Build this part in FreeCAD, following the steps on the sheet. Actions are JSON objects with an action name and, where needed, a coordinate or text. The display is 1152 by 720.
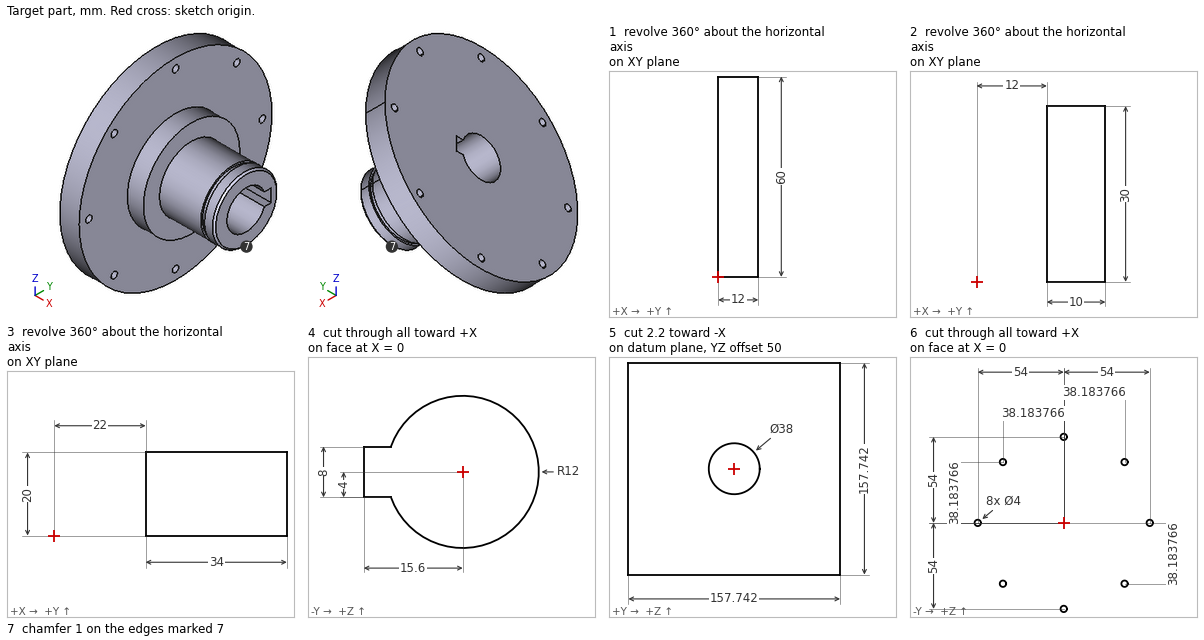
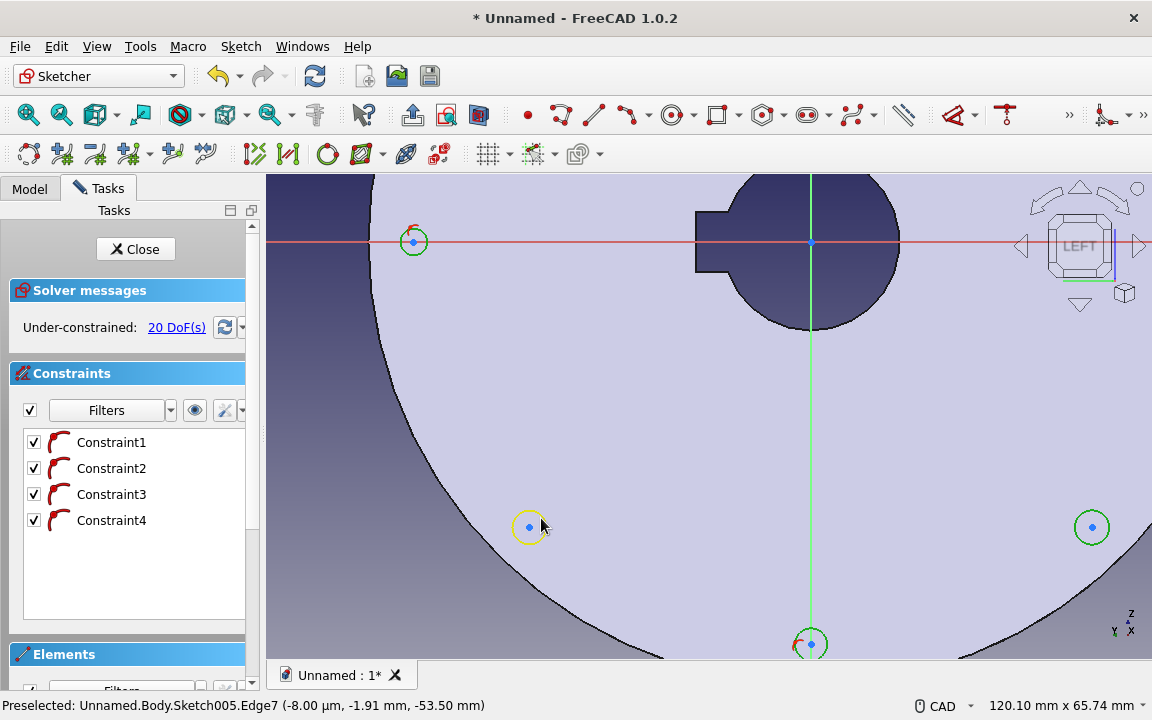
{"action": "left_click", "coordinate": [541, 516]}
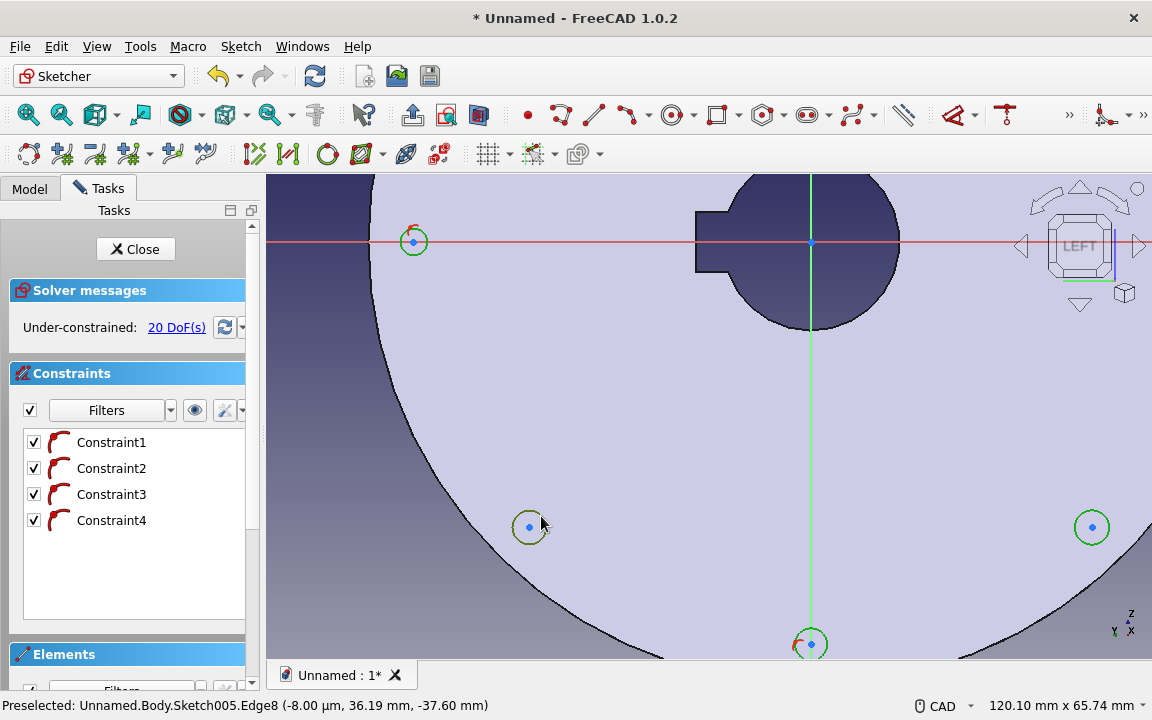
{"action": "key", "text": "e"}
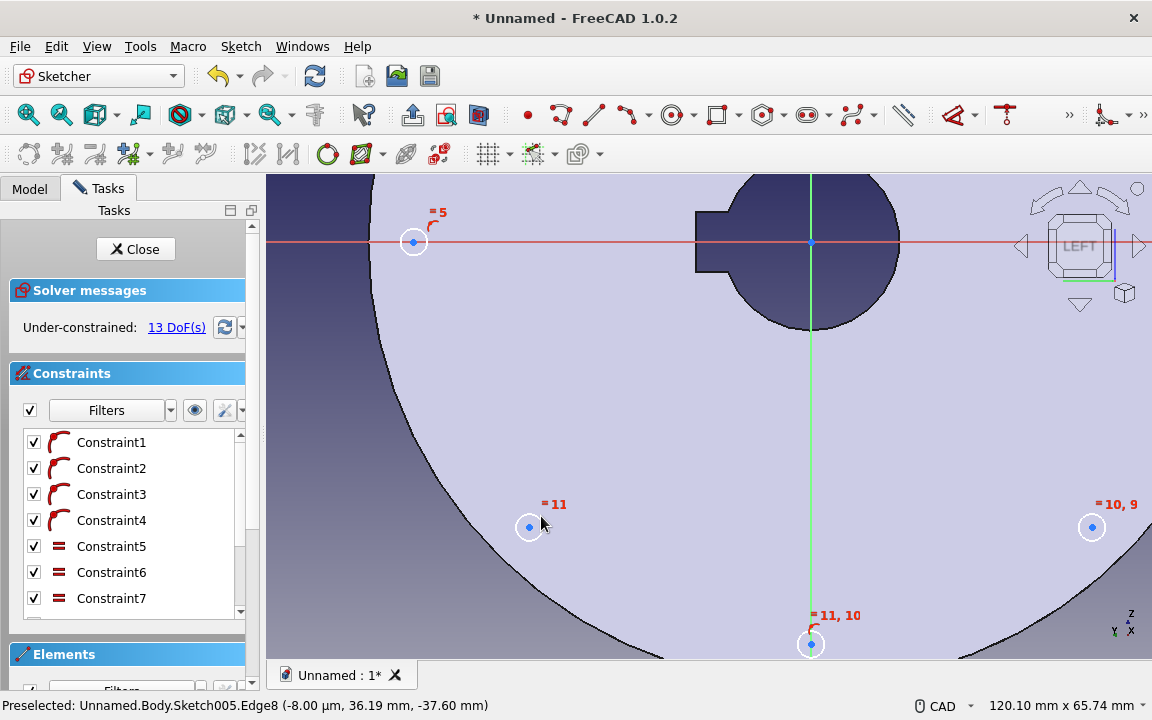
{"action": "scroll", "coordinate": [541, 518], "scroll_direction": "down", "scroll_amount": 5}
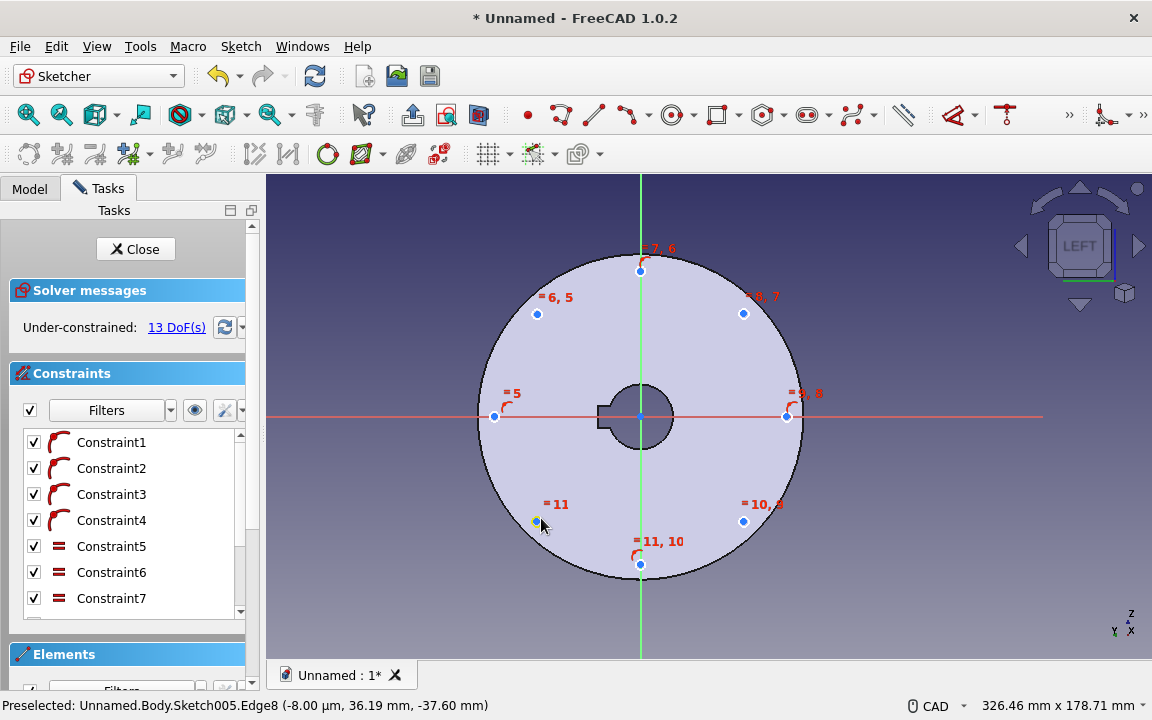
{"action": "left_click", "coordinate": [537, 314]}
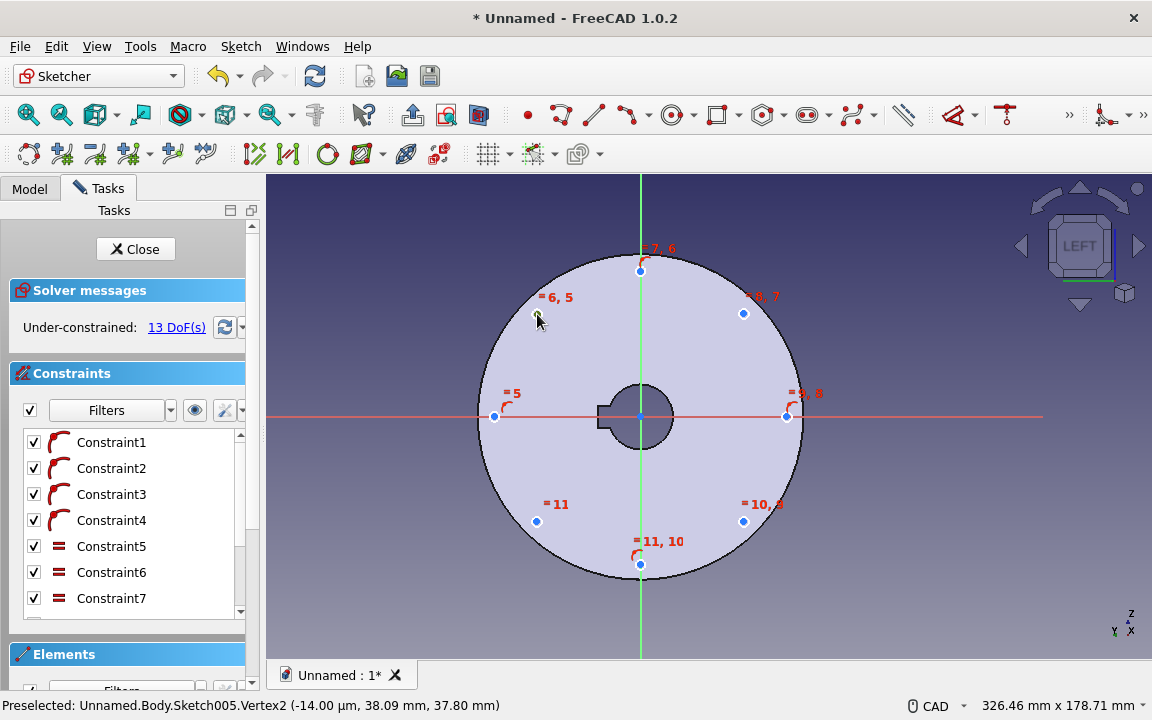
{"action": "left_click", "coordinate": [744, 314]}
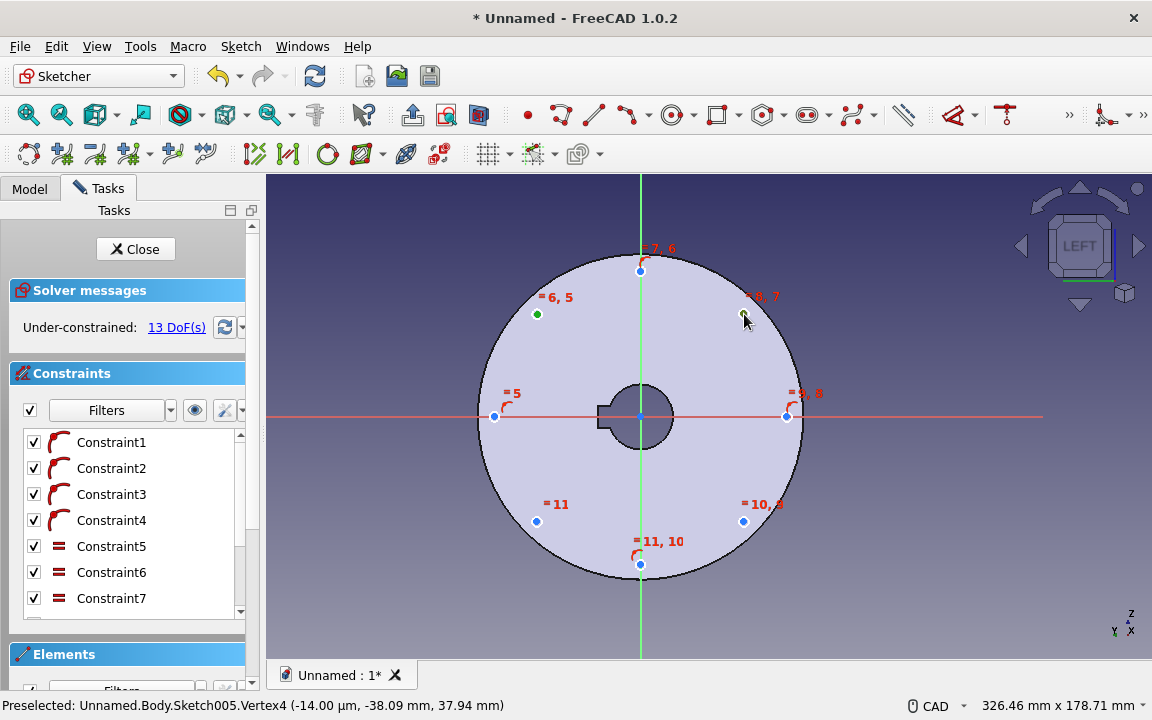
{"action": "key", "text": "h"}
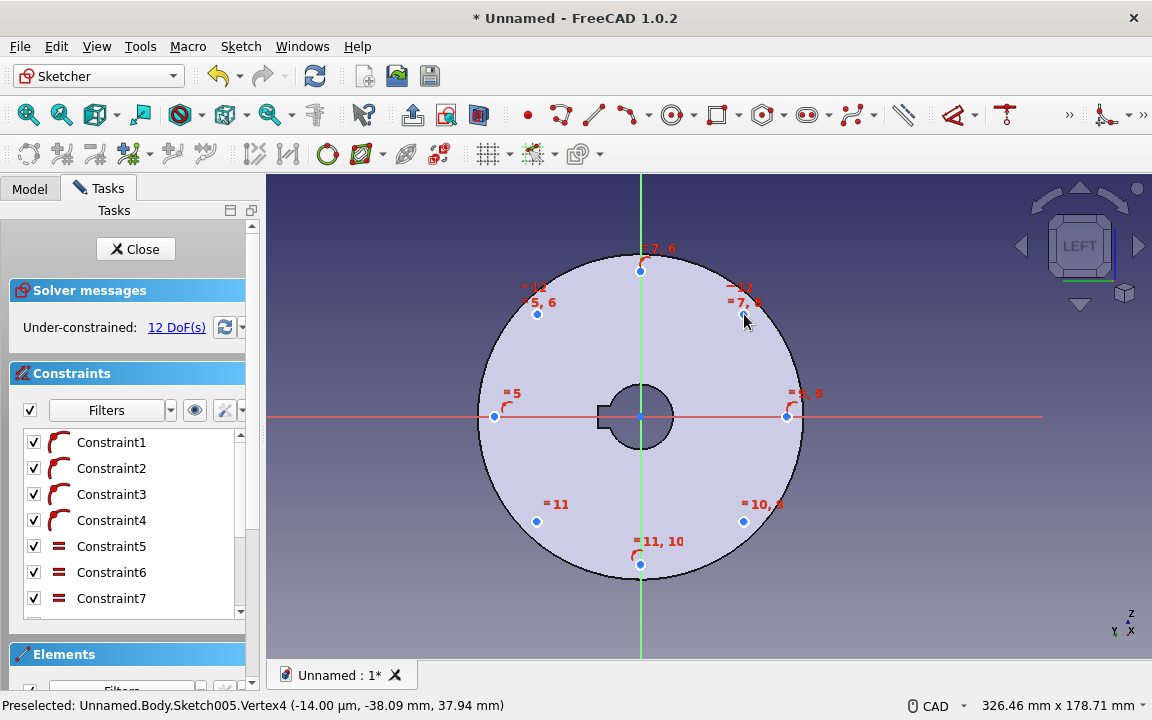
{"action": "left_click", "coordinate": [744, 314]}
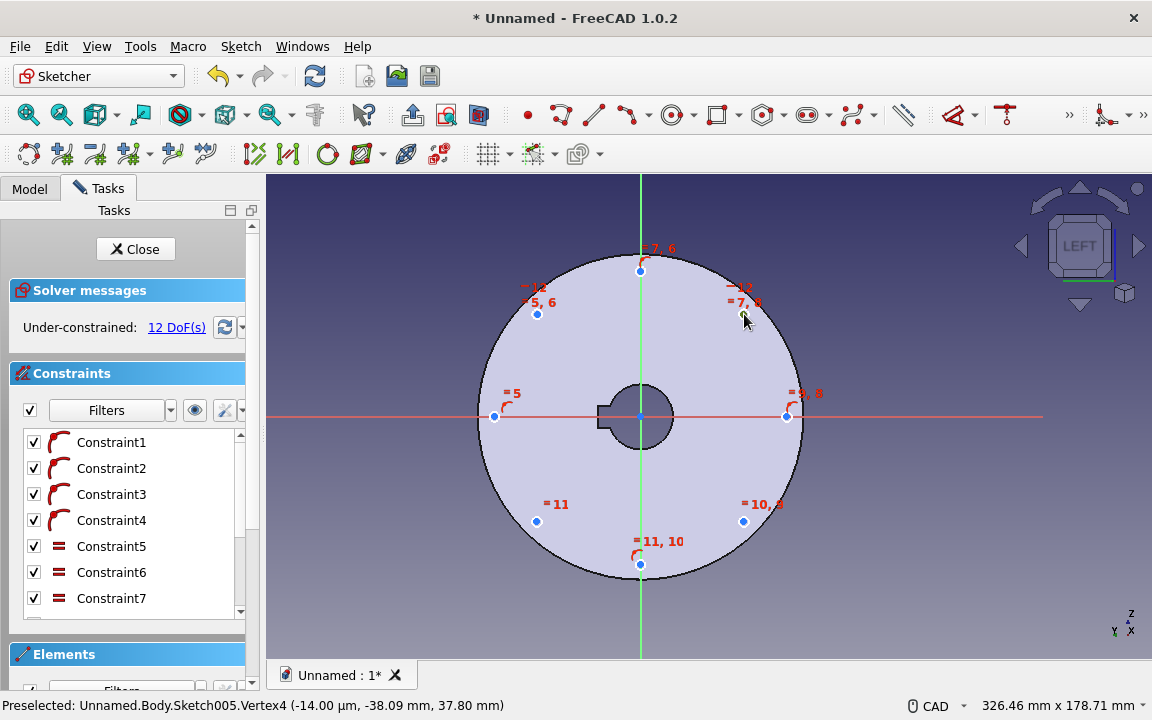
{"action": "left_click", "coordinate": [744, 522]}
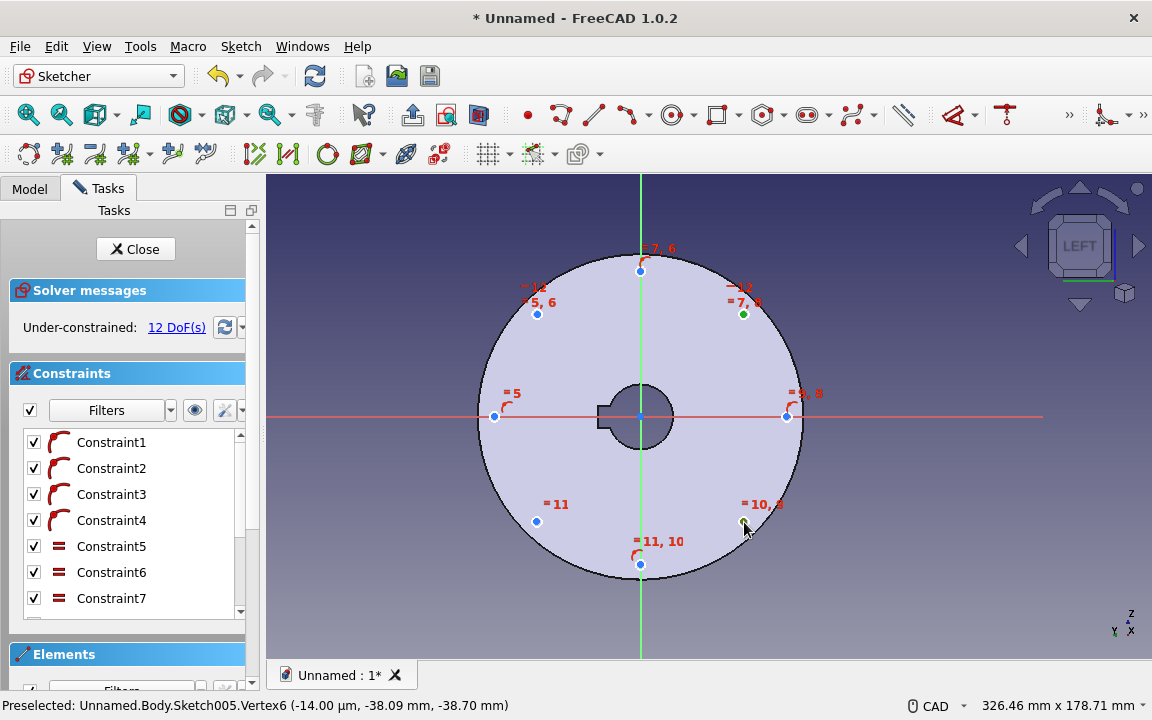
{"action": "key", "text": "v"}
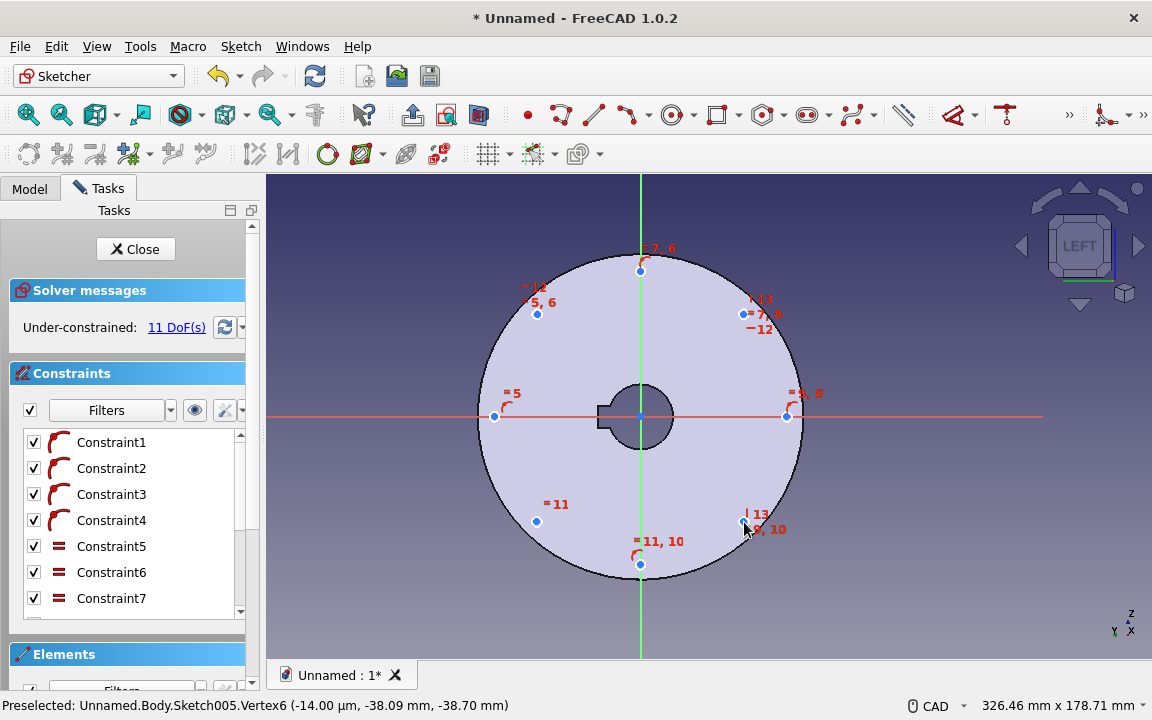
{"action": "left_click", "coordinate": [537, 314]}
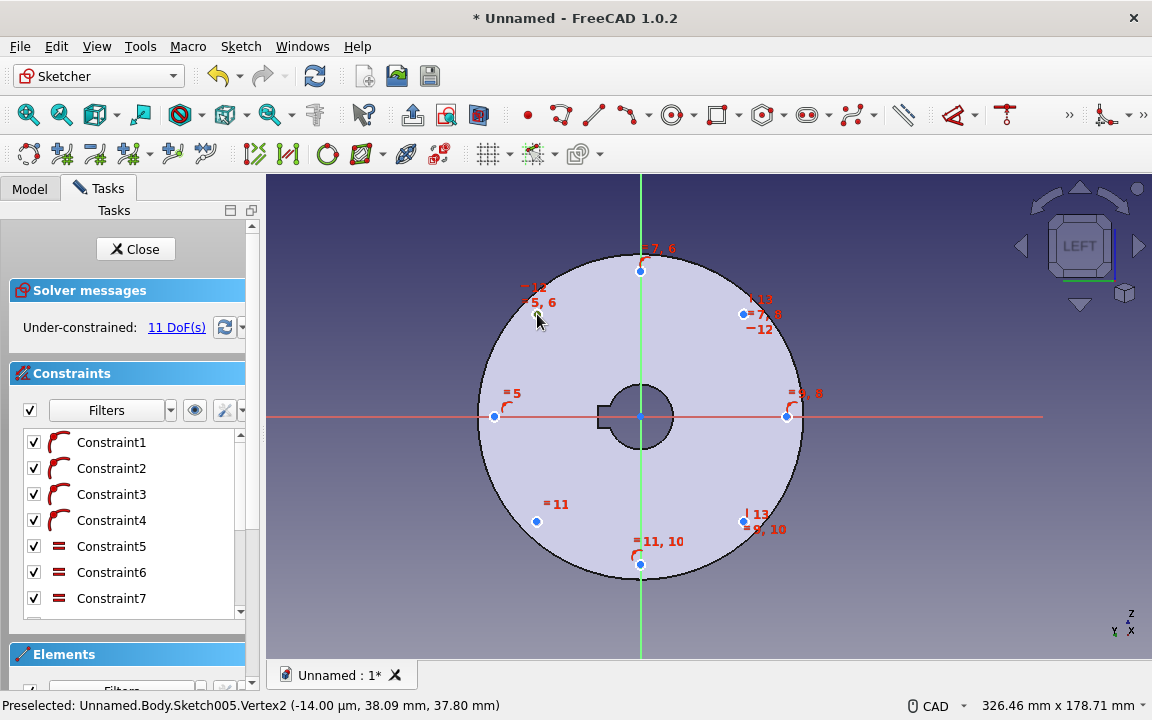
{"action": "left_click", "coordinate": [537, 522]}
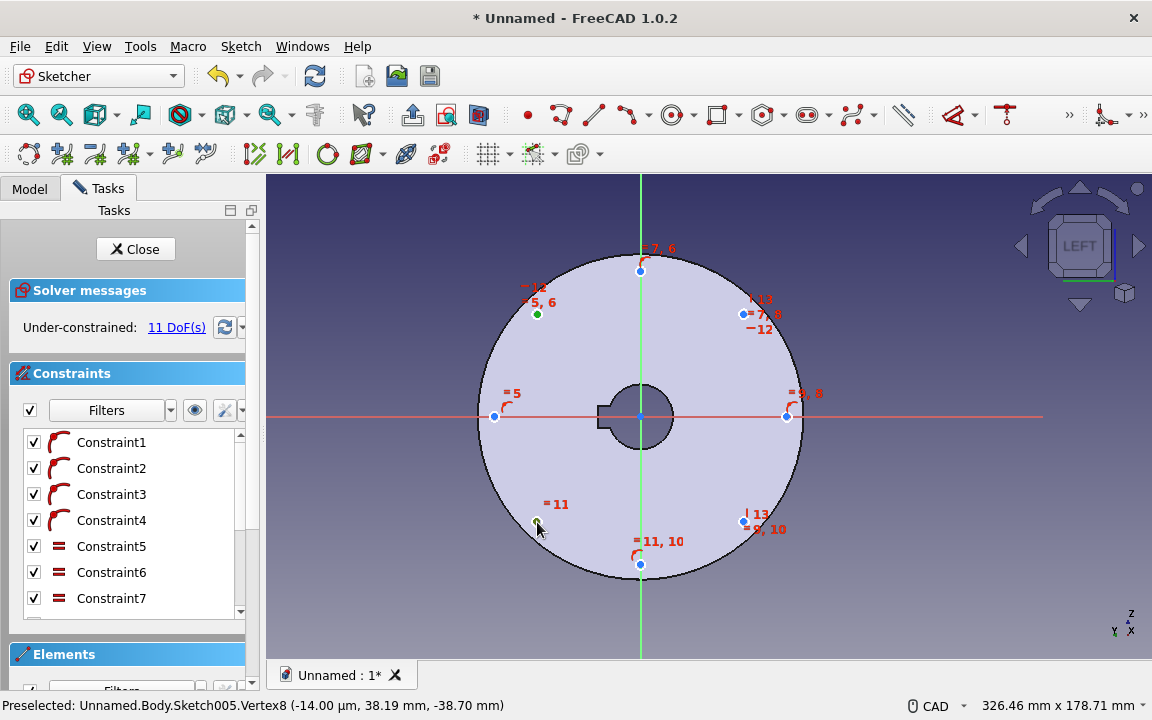
{"action": "key", "text": "v"}